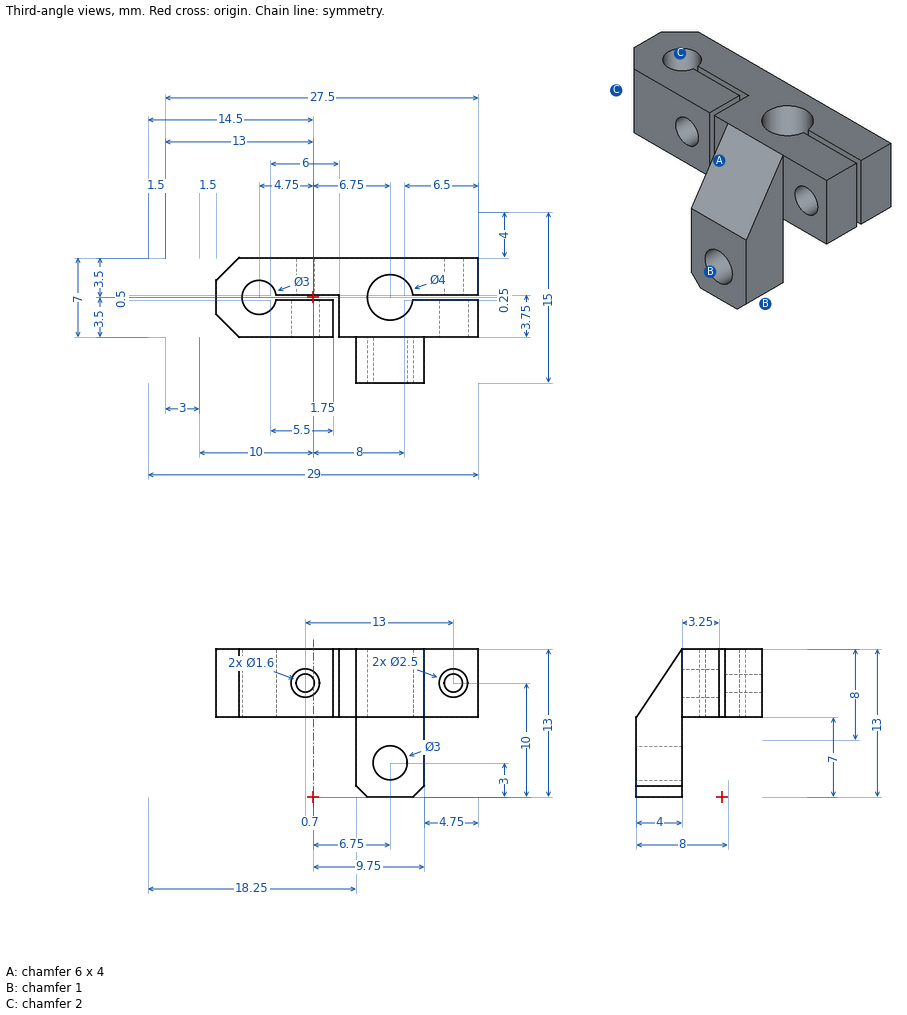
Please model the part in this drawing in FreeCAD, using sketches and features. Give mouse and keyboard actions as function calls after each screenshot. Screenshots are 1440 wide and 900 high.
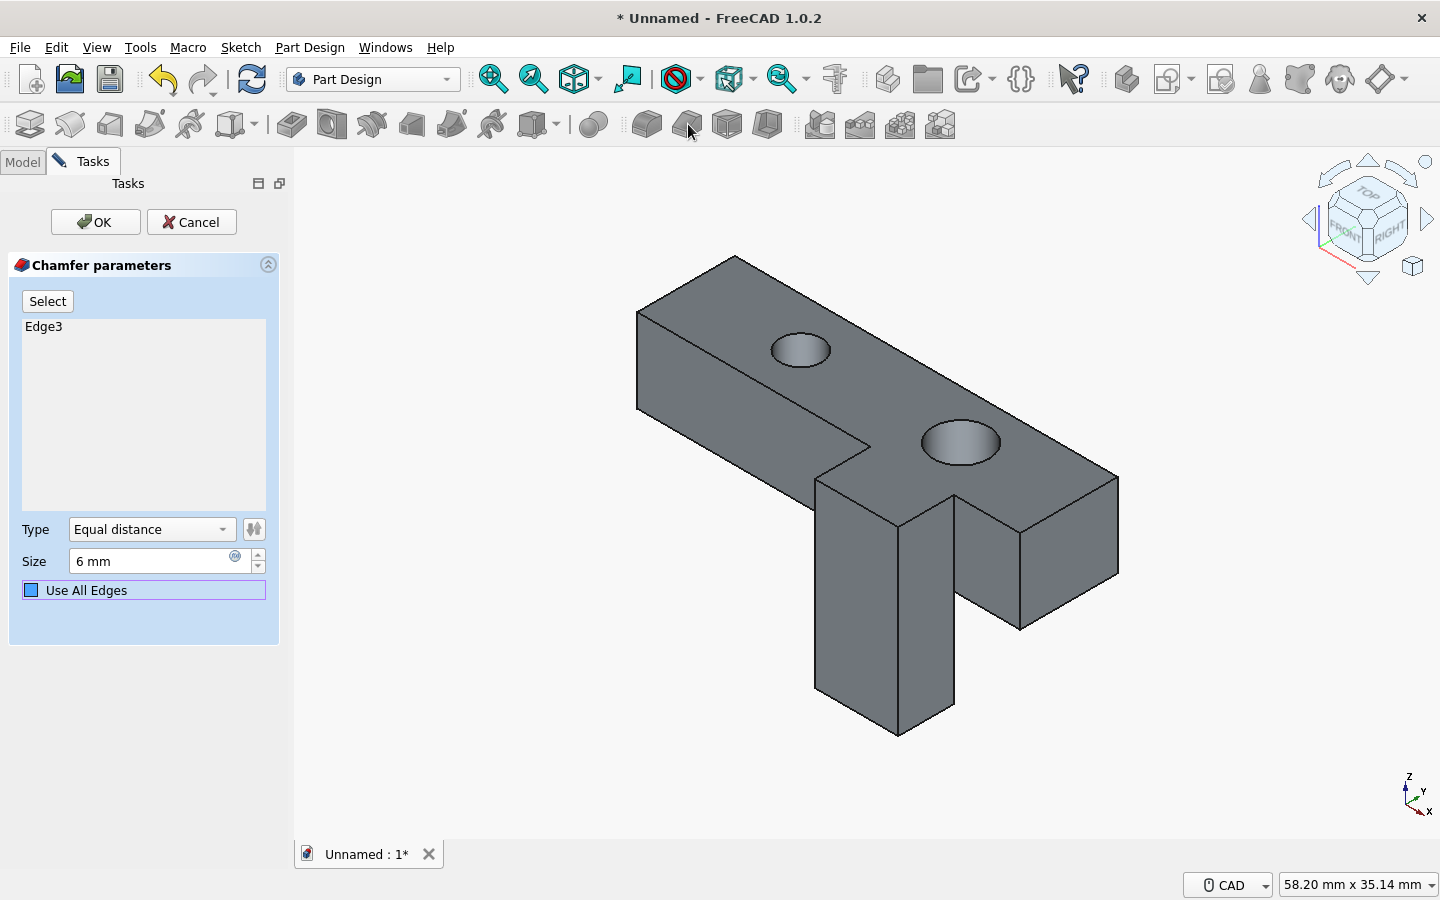
click(153, 530)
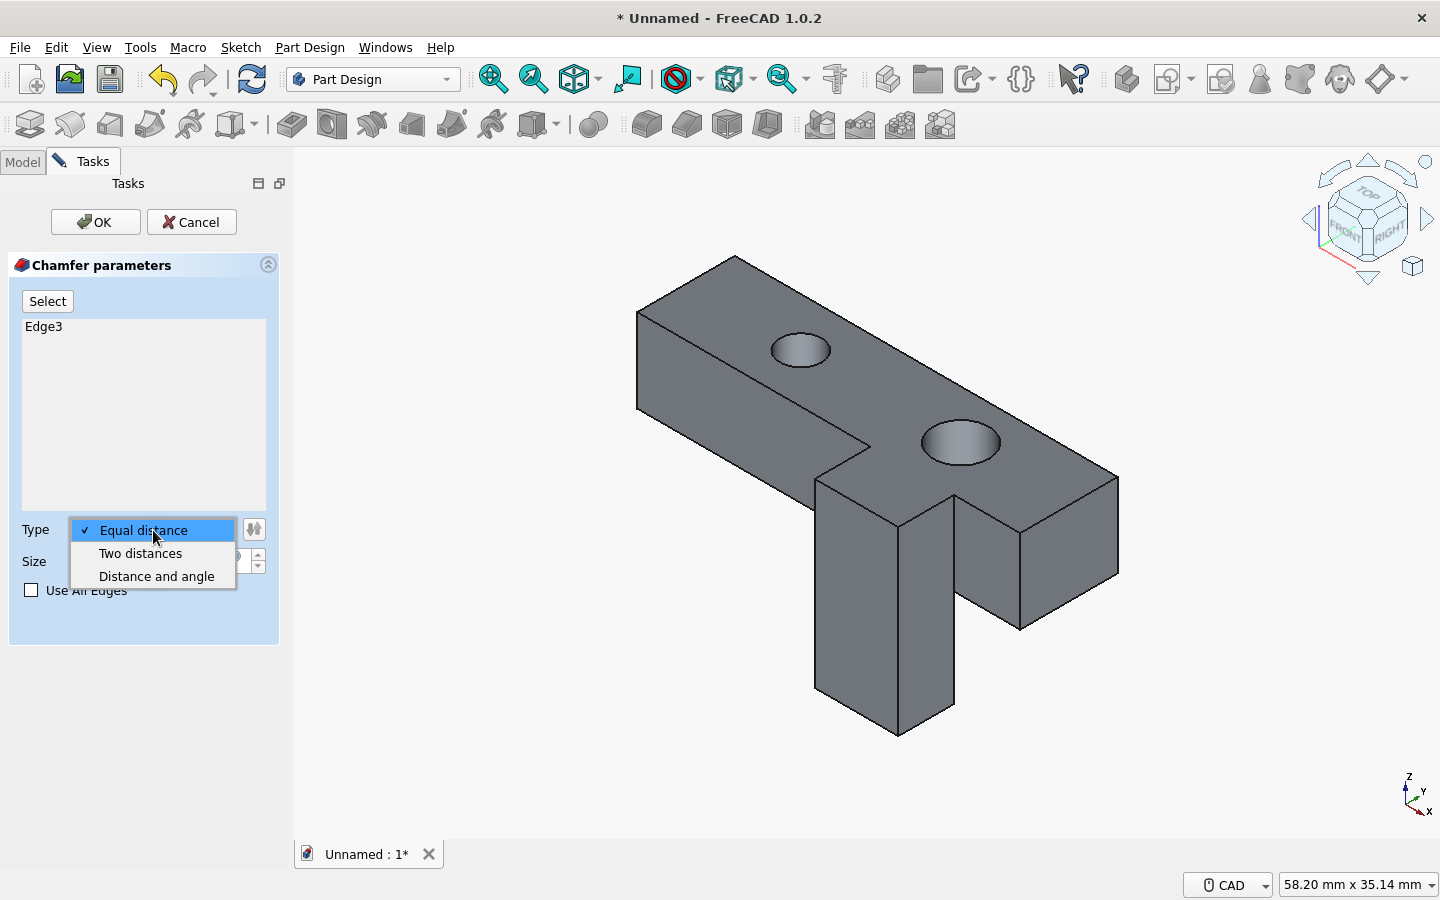
click(152, 554)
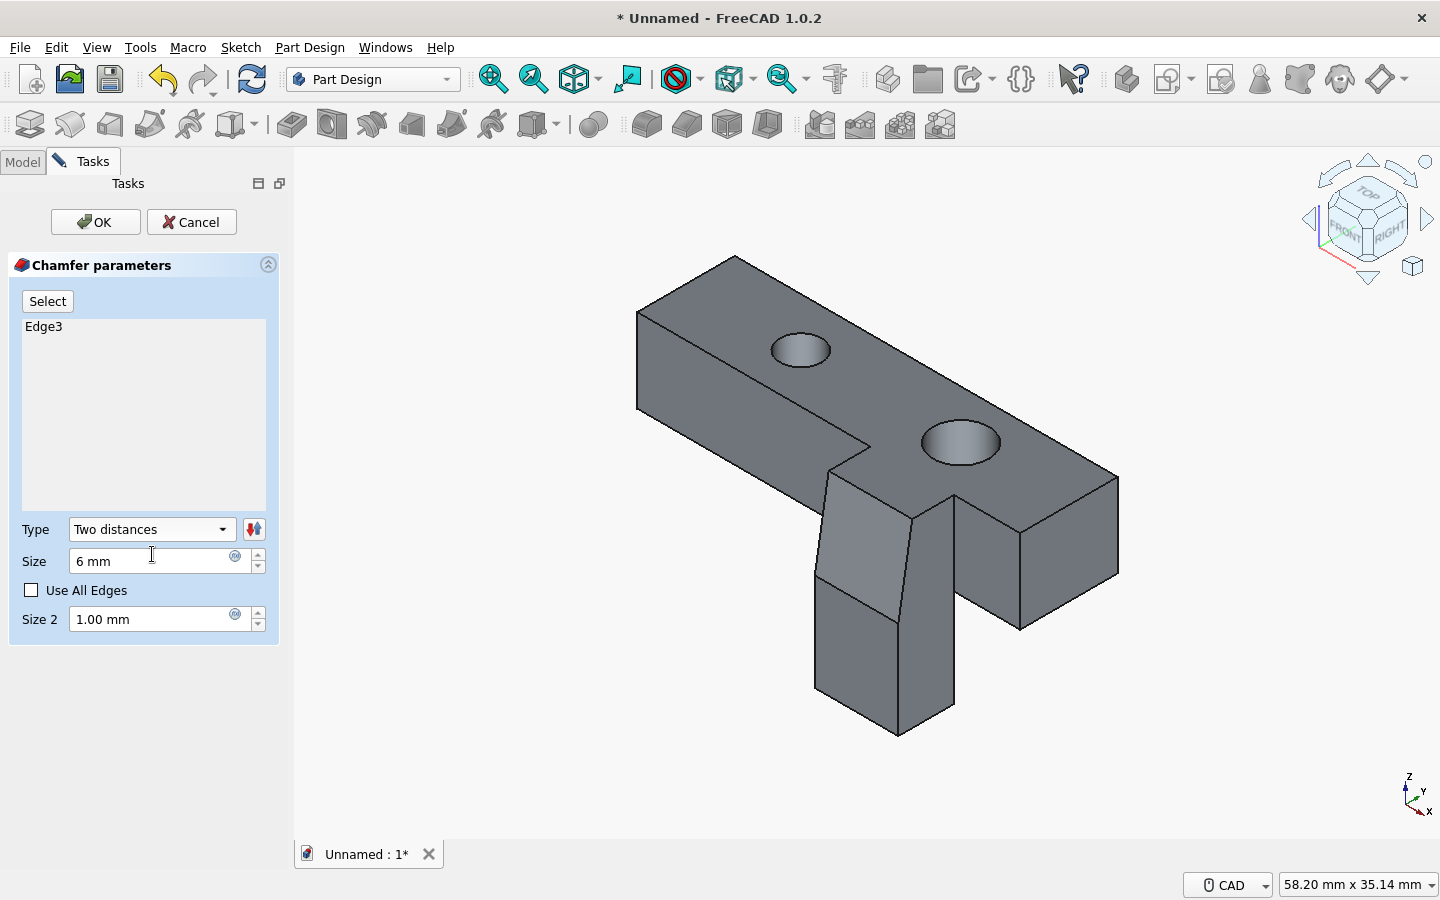
triple_click(160, 619)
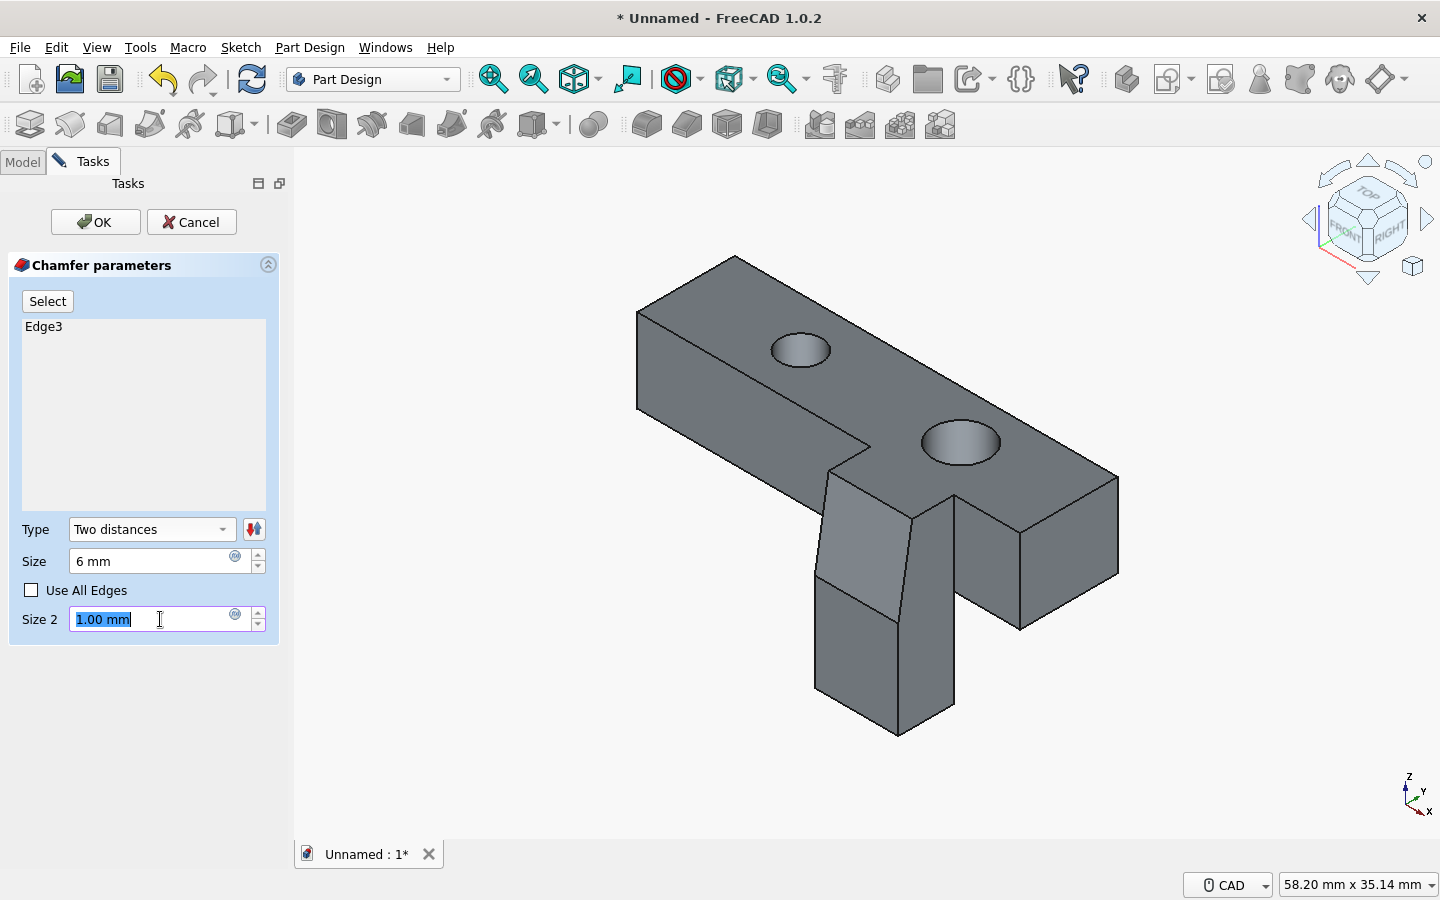
text(4)
key(Tab)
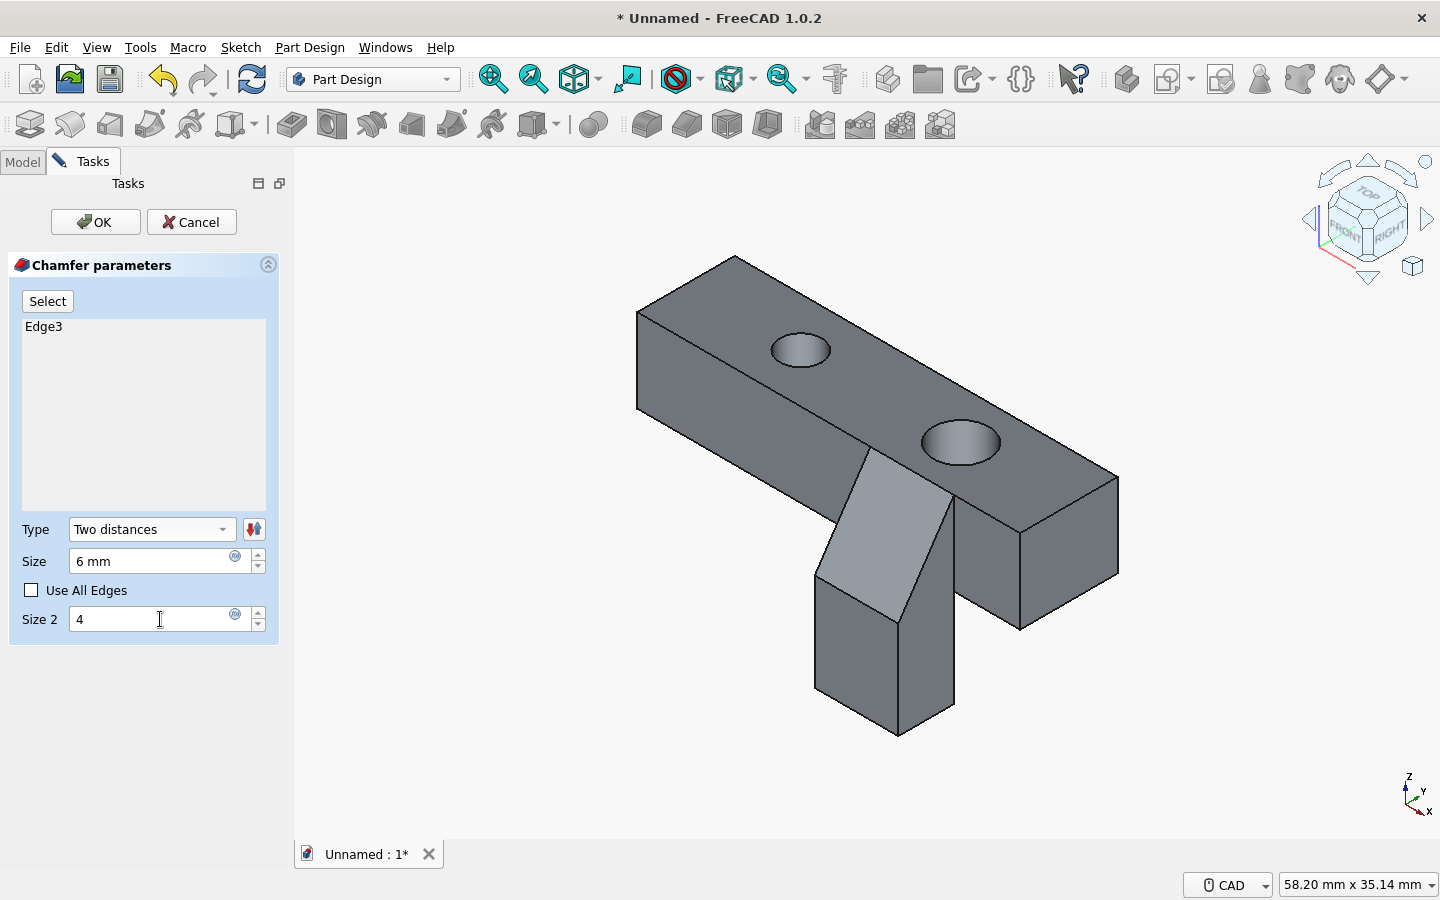
click(96, 222)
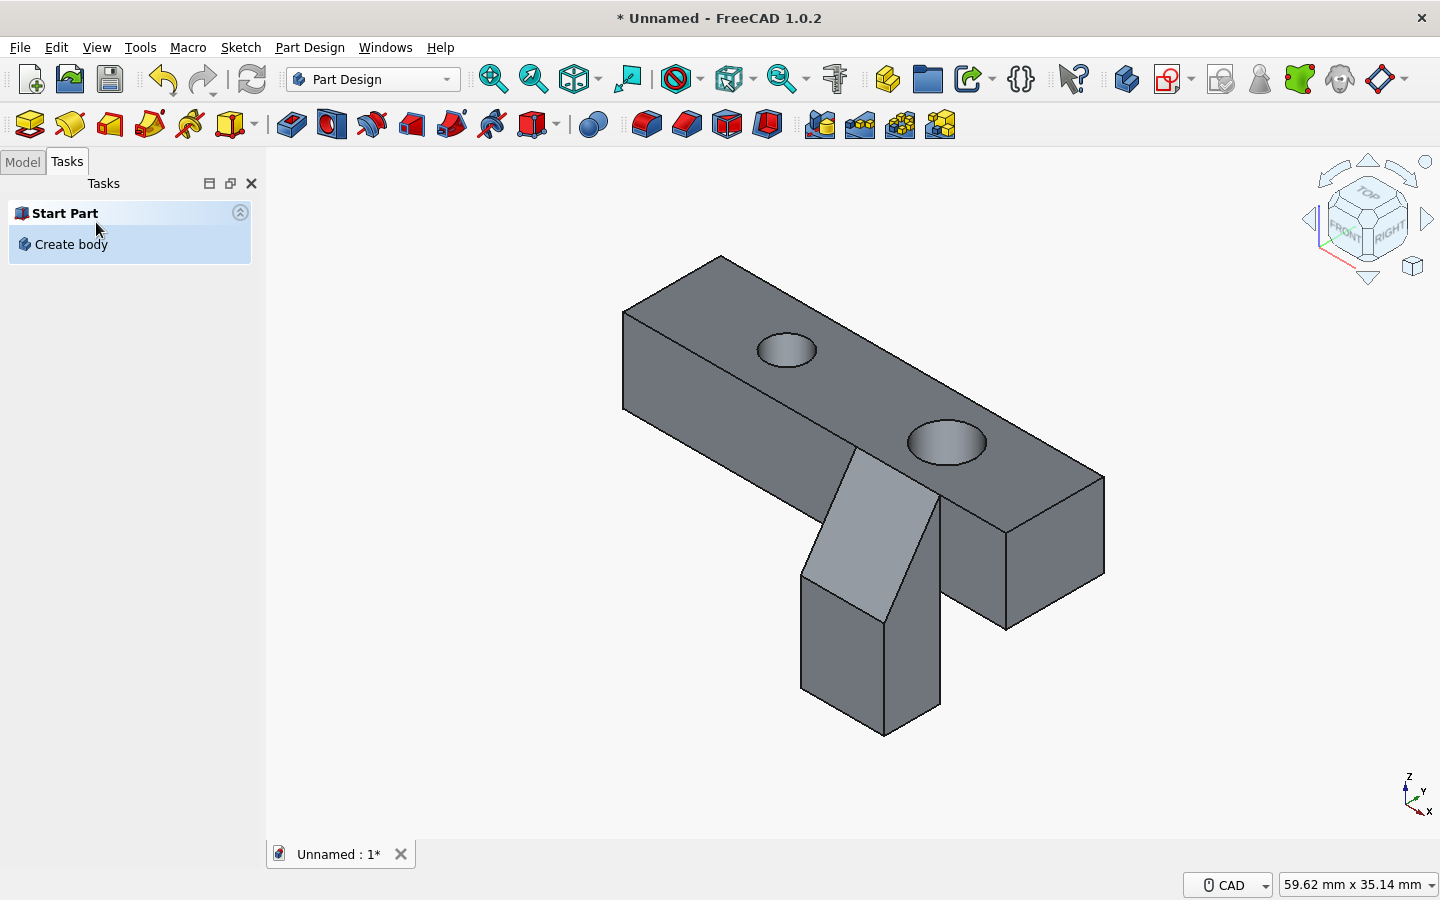
key(5)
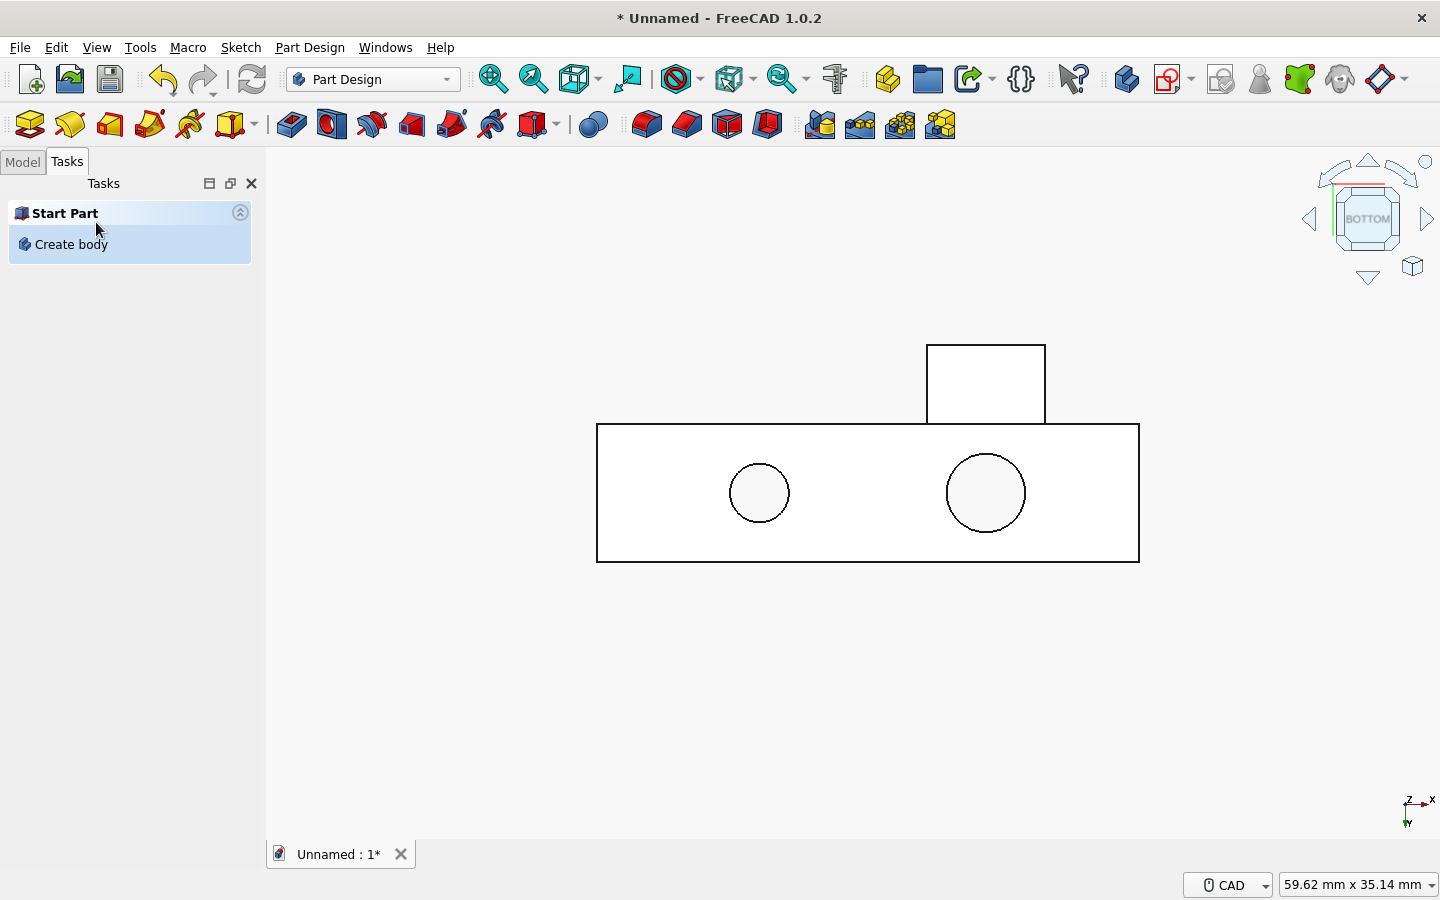
click(868, 492)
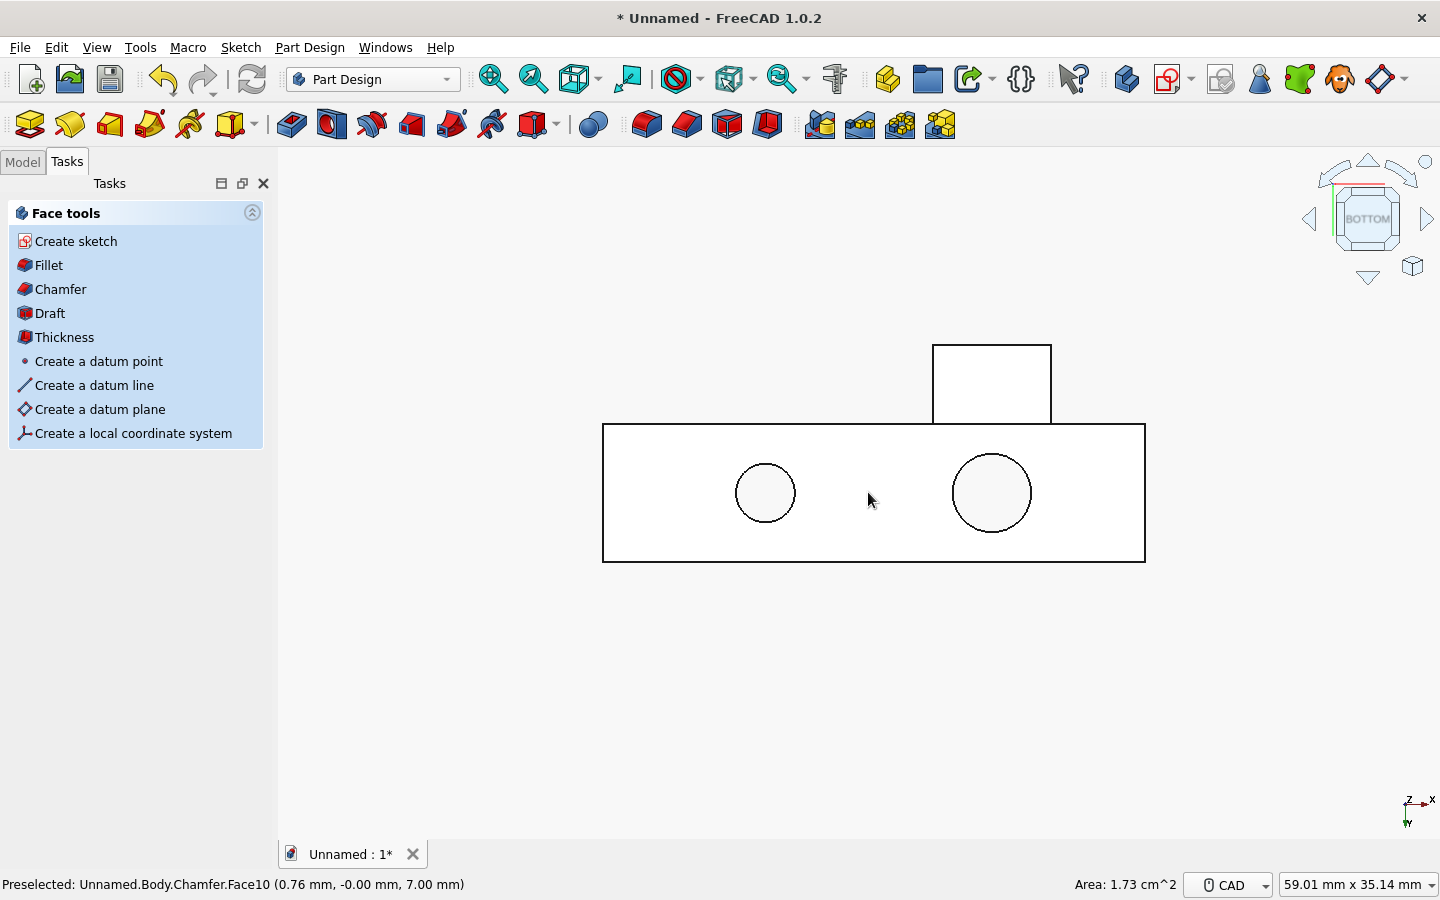
click(1168, 80)